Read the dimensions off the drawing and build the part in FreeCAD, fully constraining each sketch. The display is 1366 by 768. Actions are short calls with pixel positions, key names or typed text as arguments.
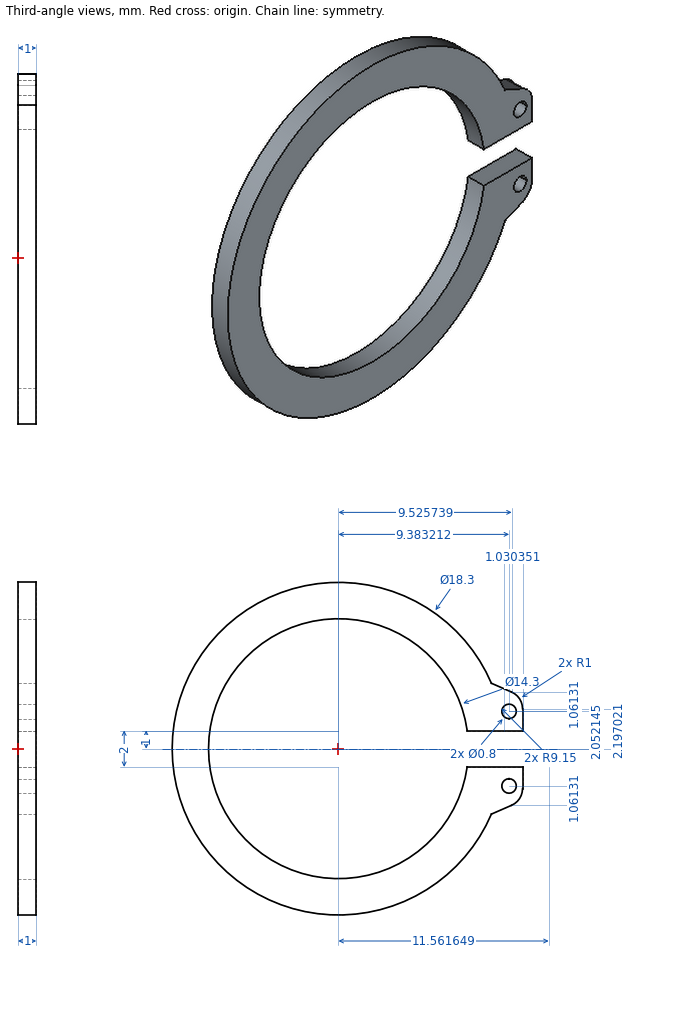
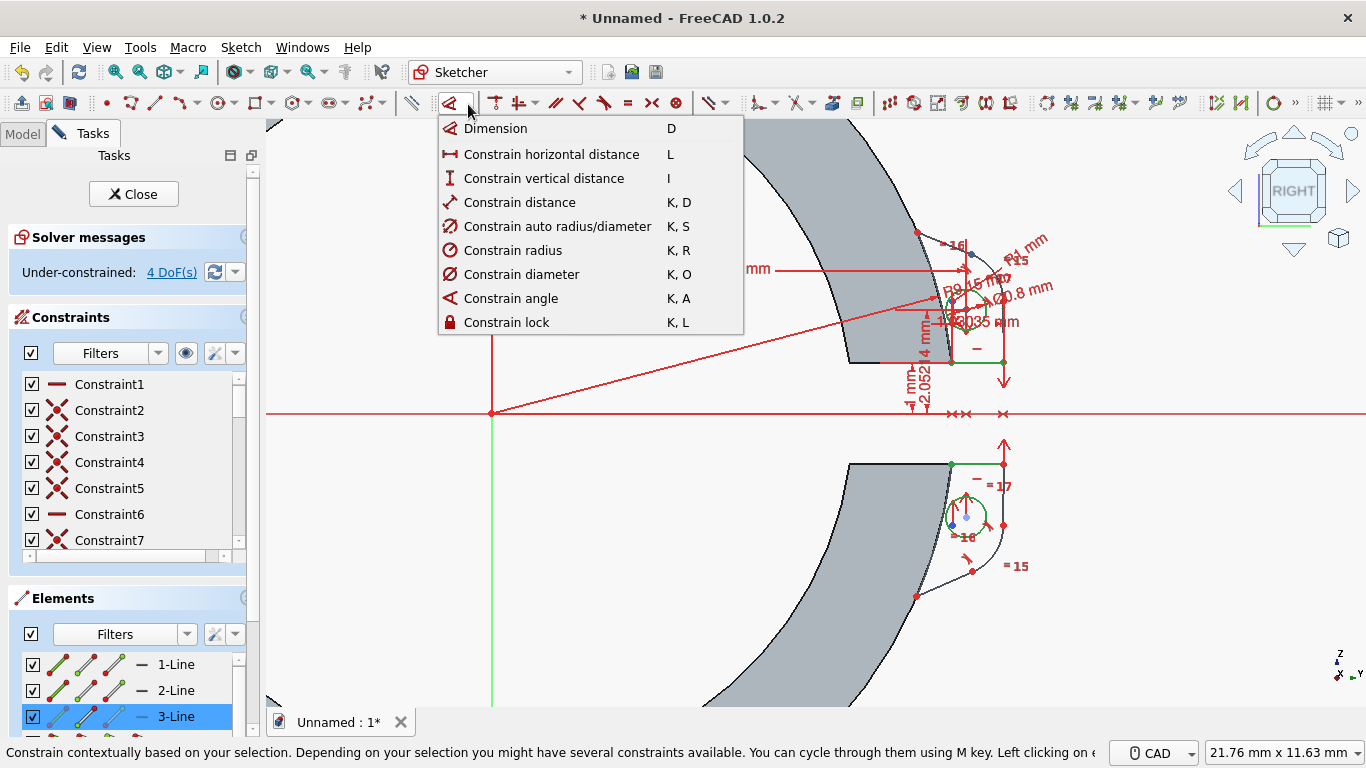
click(591, 178)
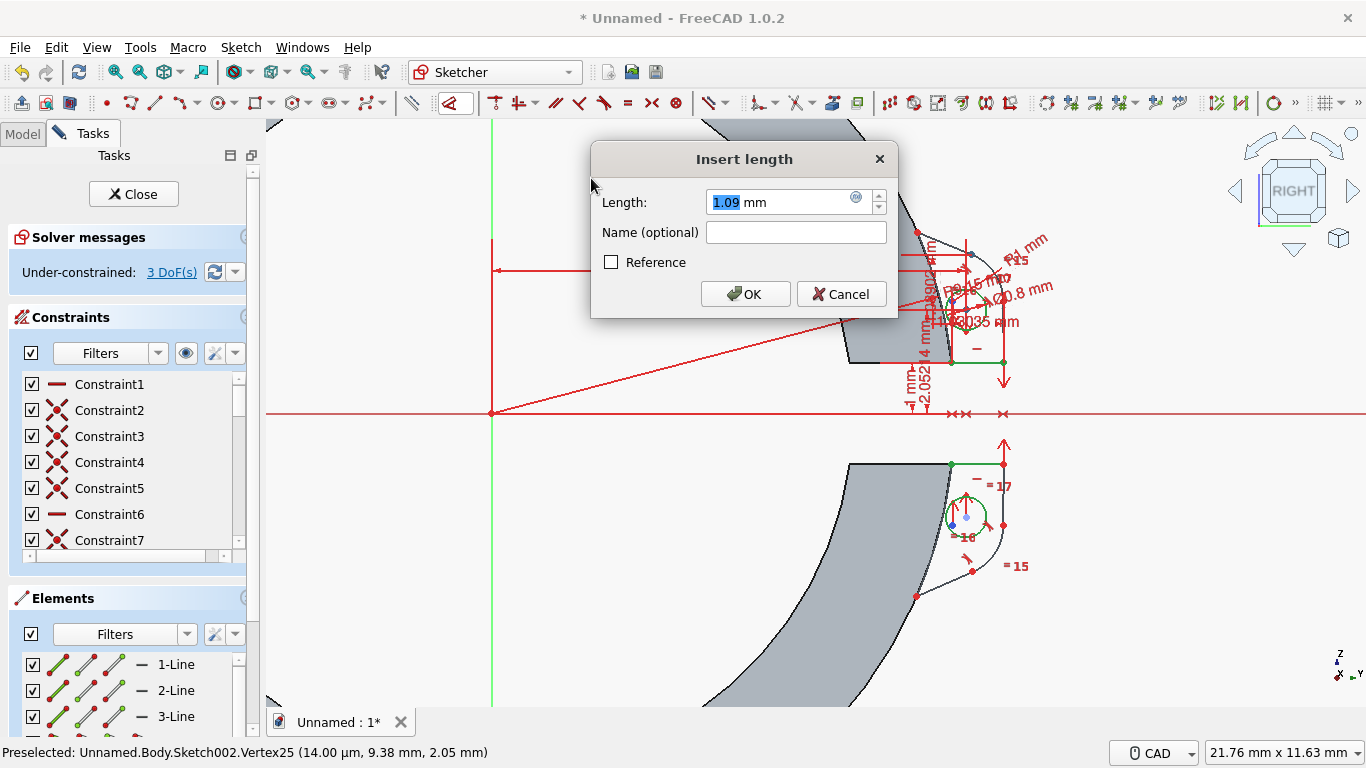
text(1.06131)
key(Return)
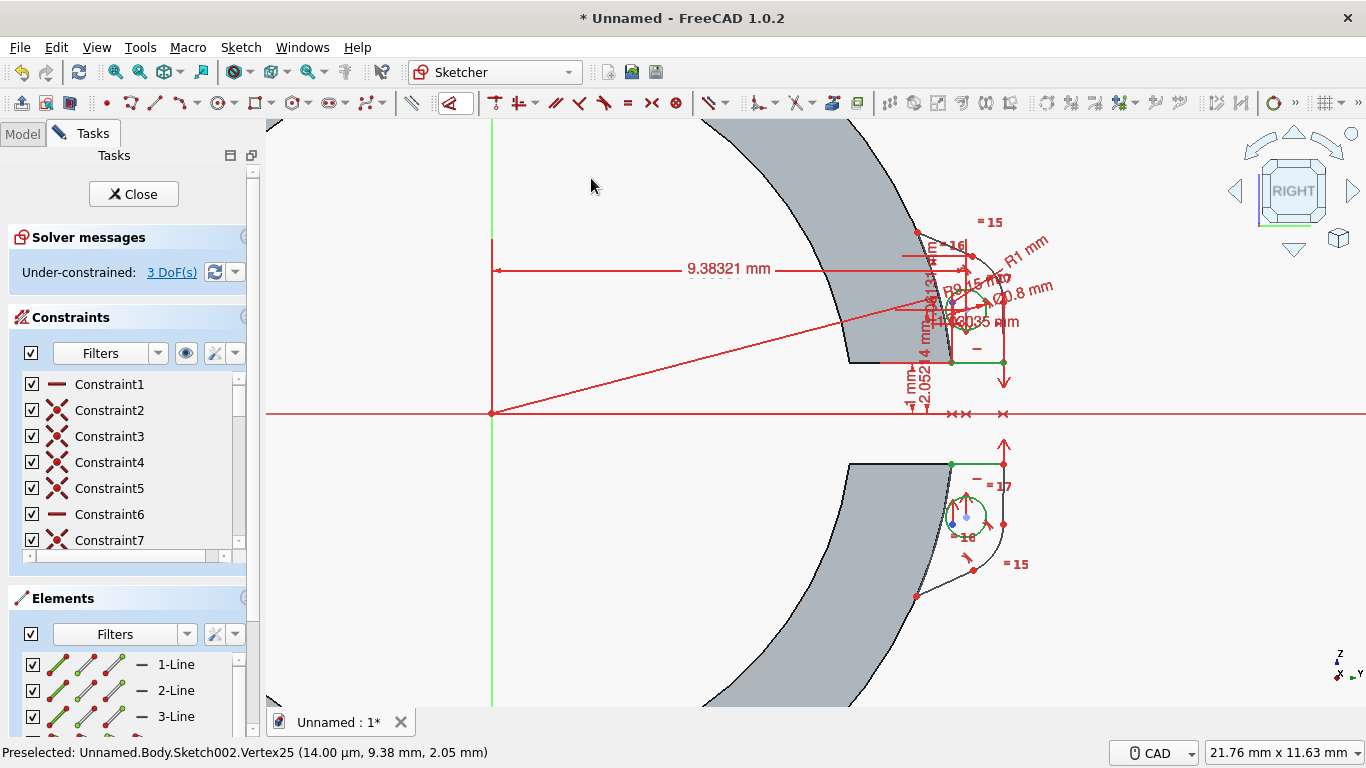
click(974, 570)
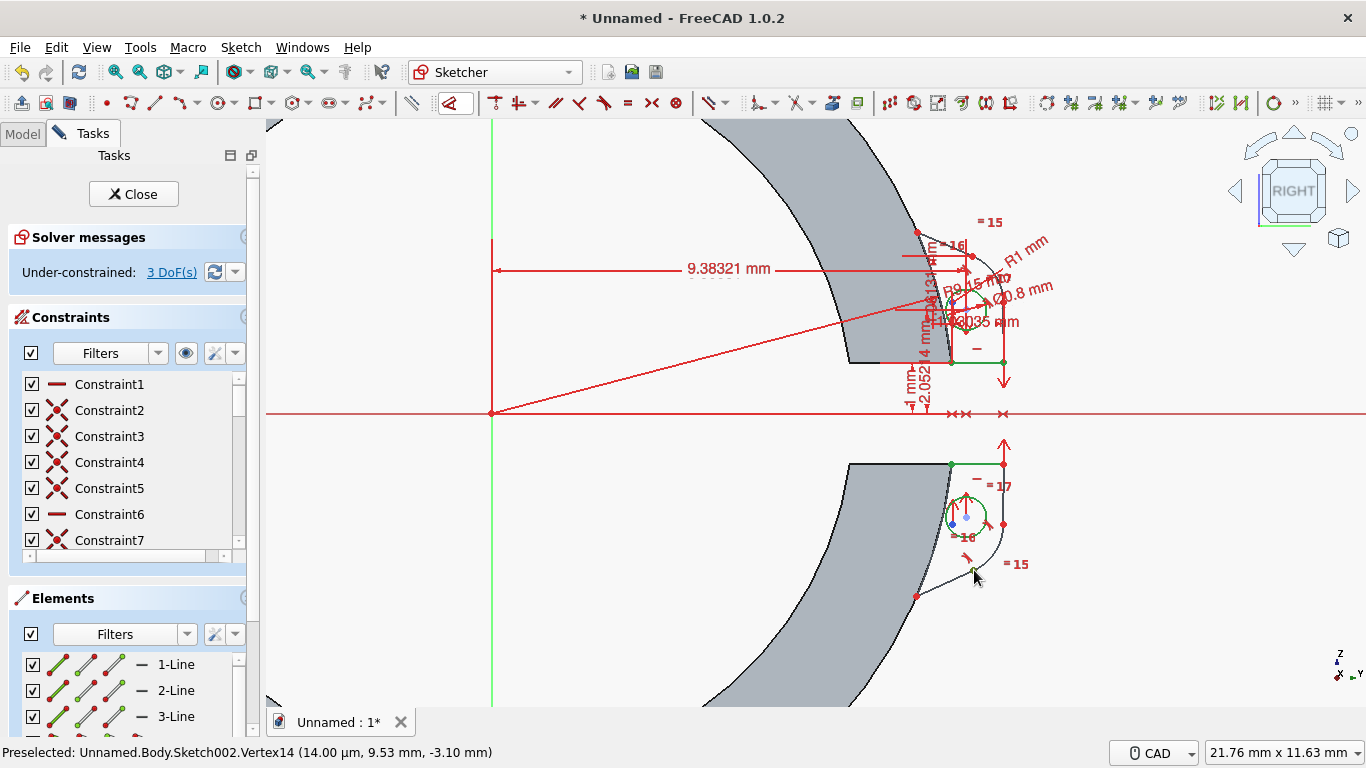
click(966, 517)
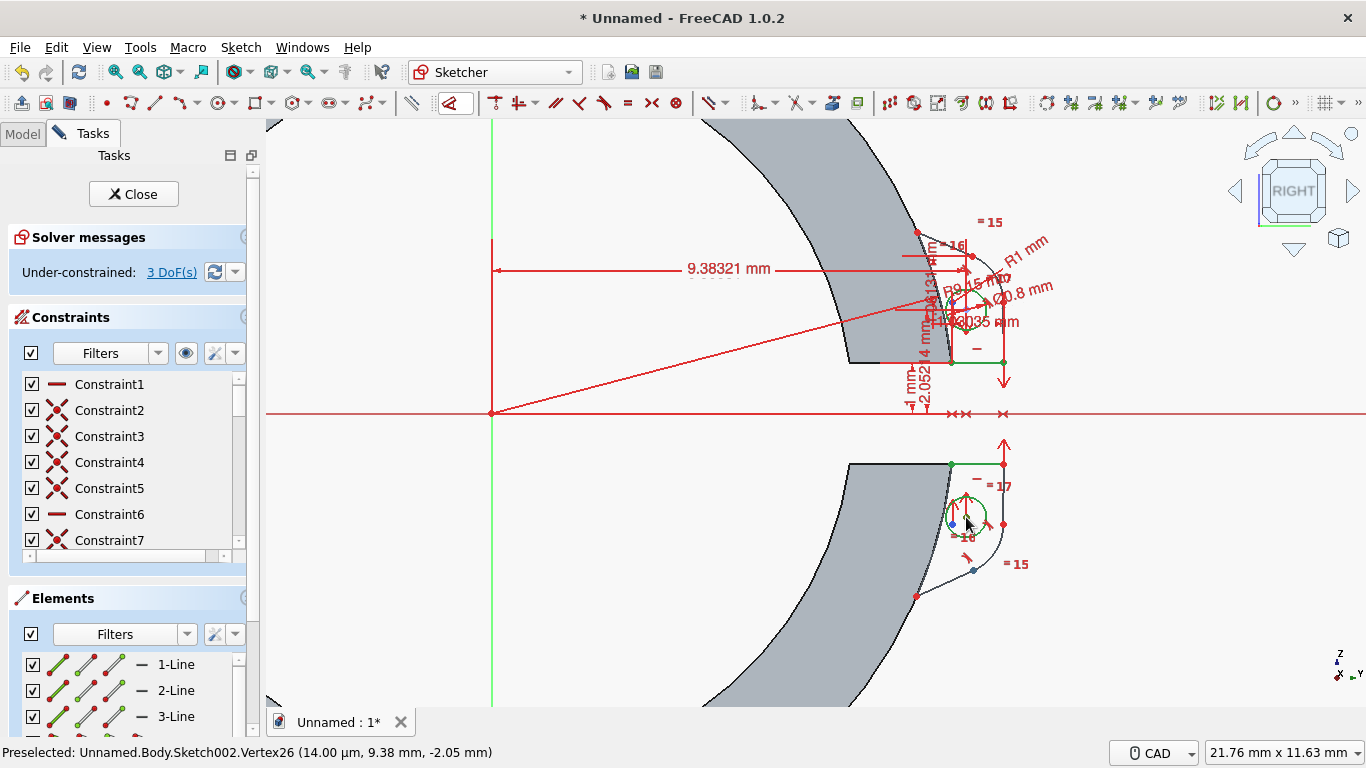
click(468, 104)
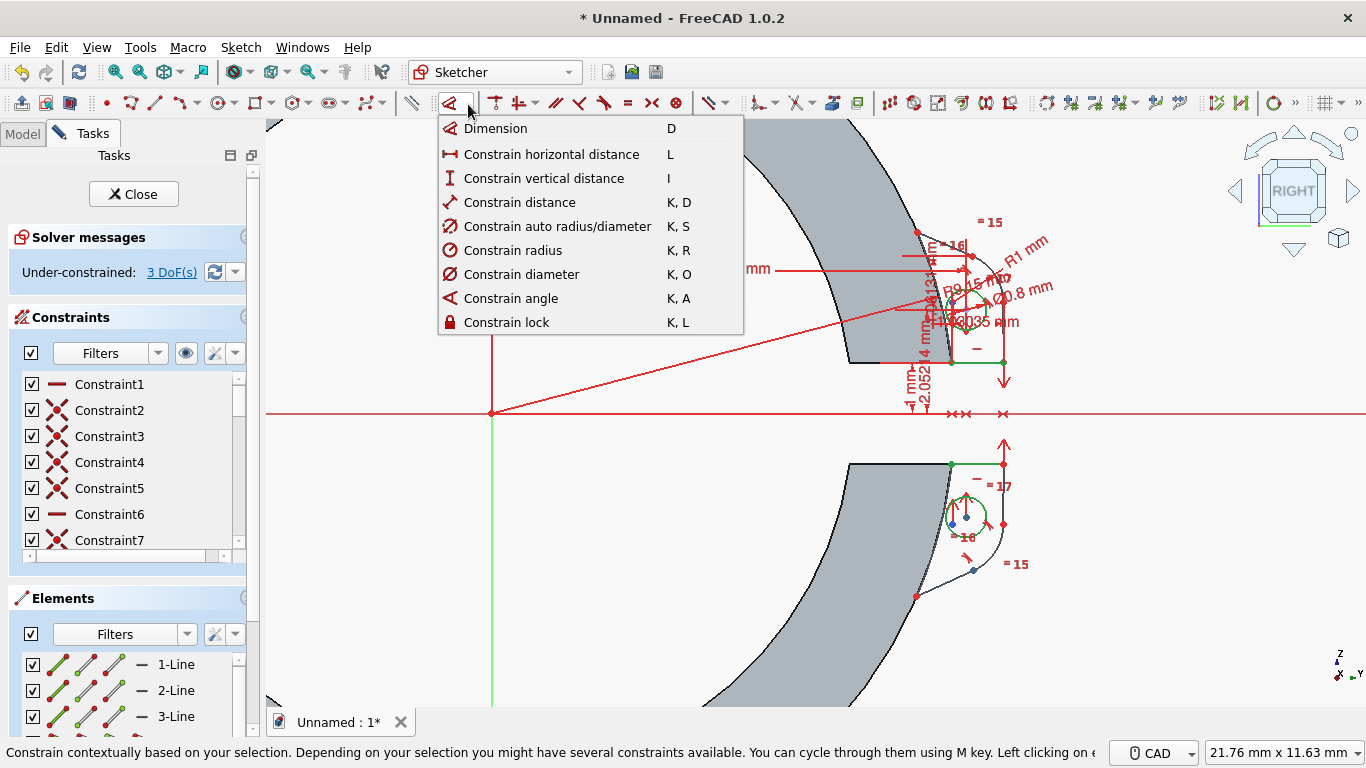
click(591, 178)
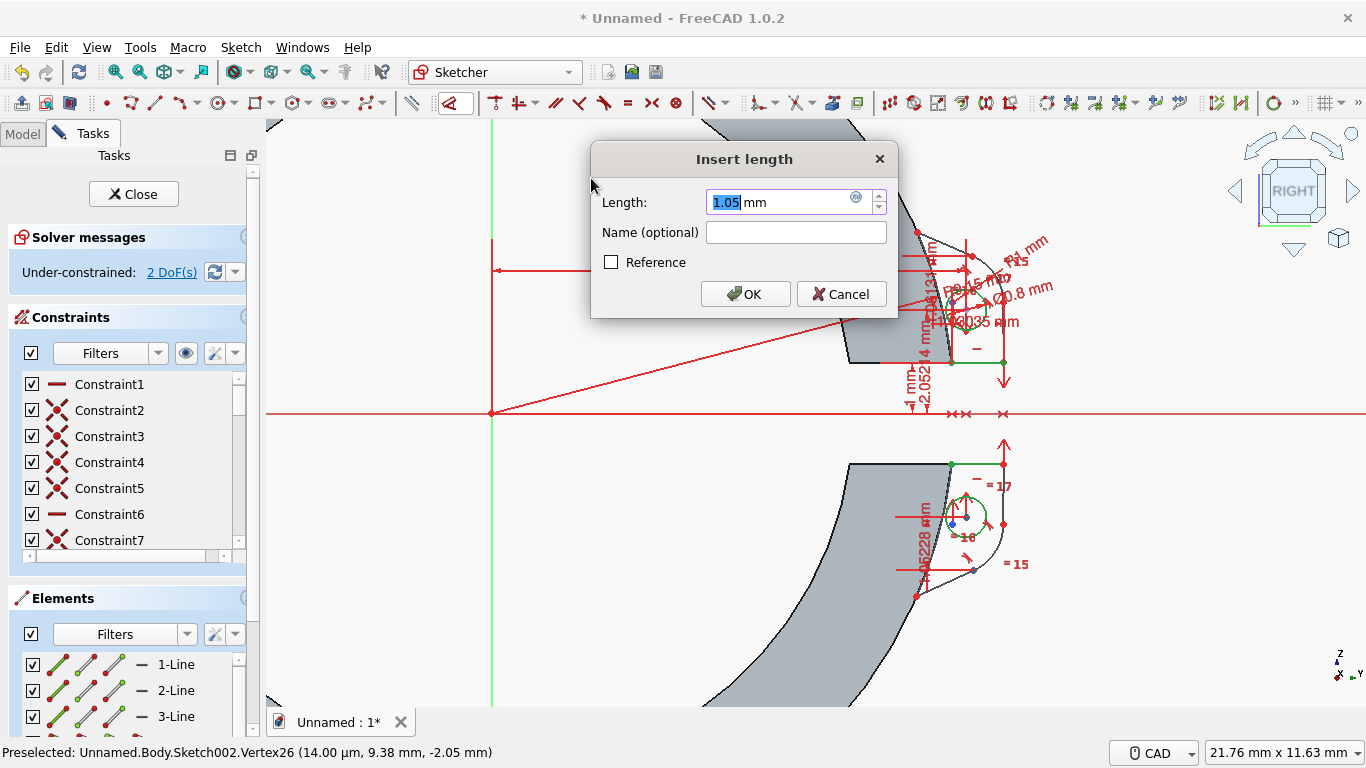
text(1.06131)
key(Return)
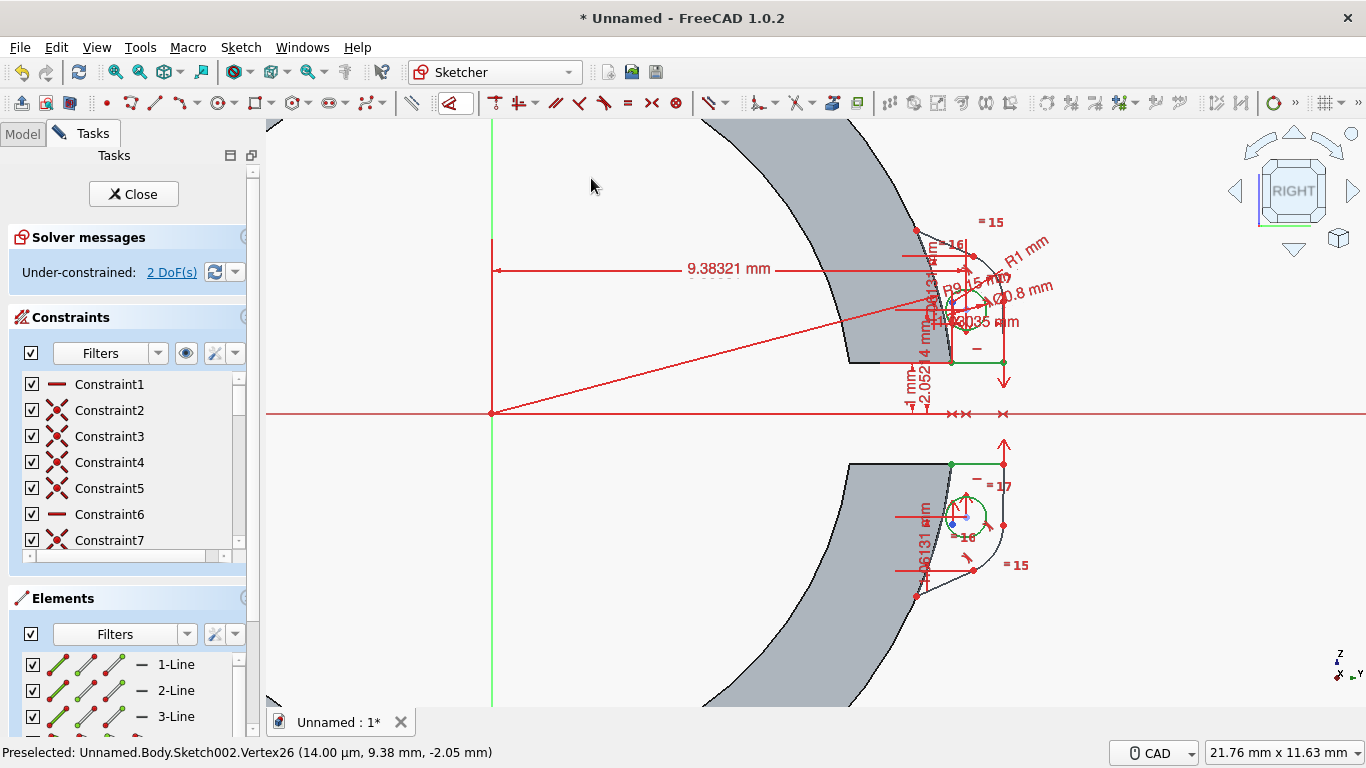
click(1003, 302)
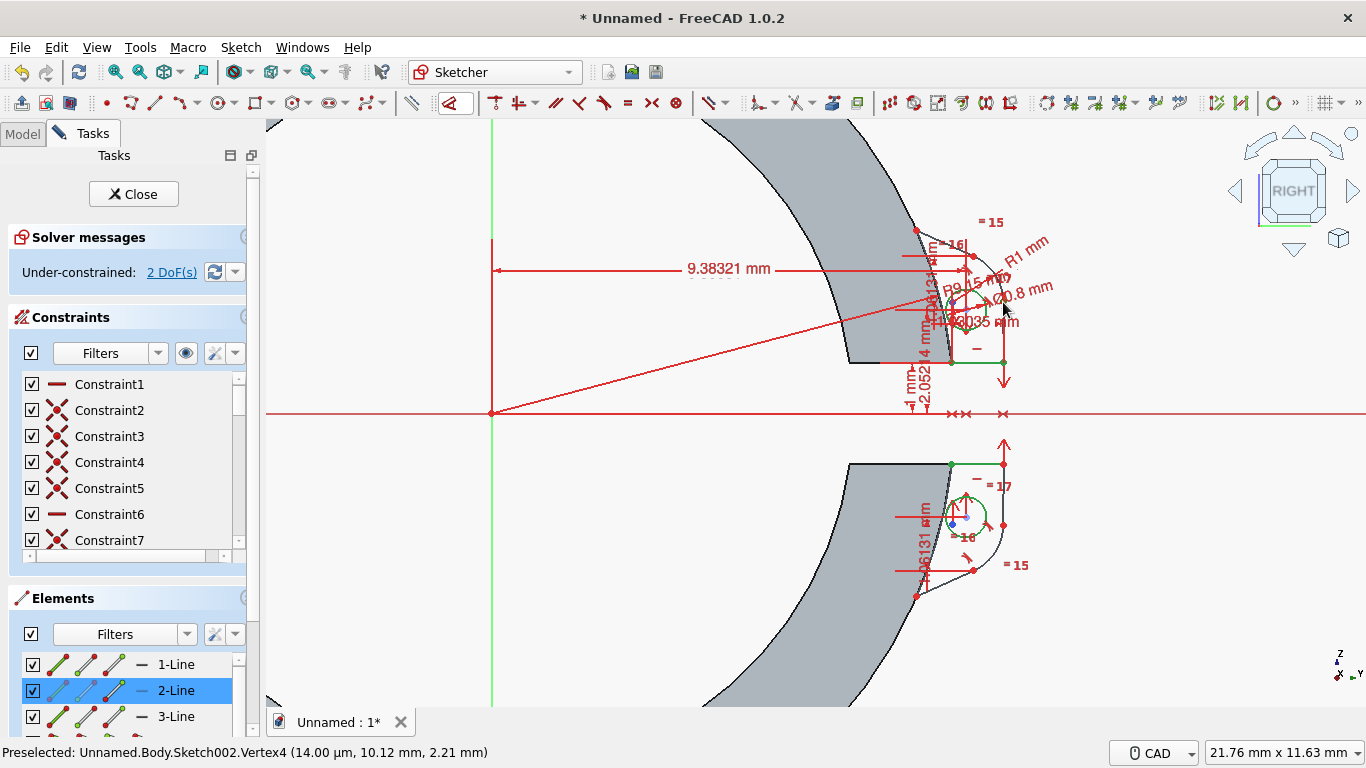
key(i)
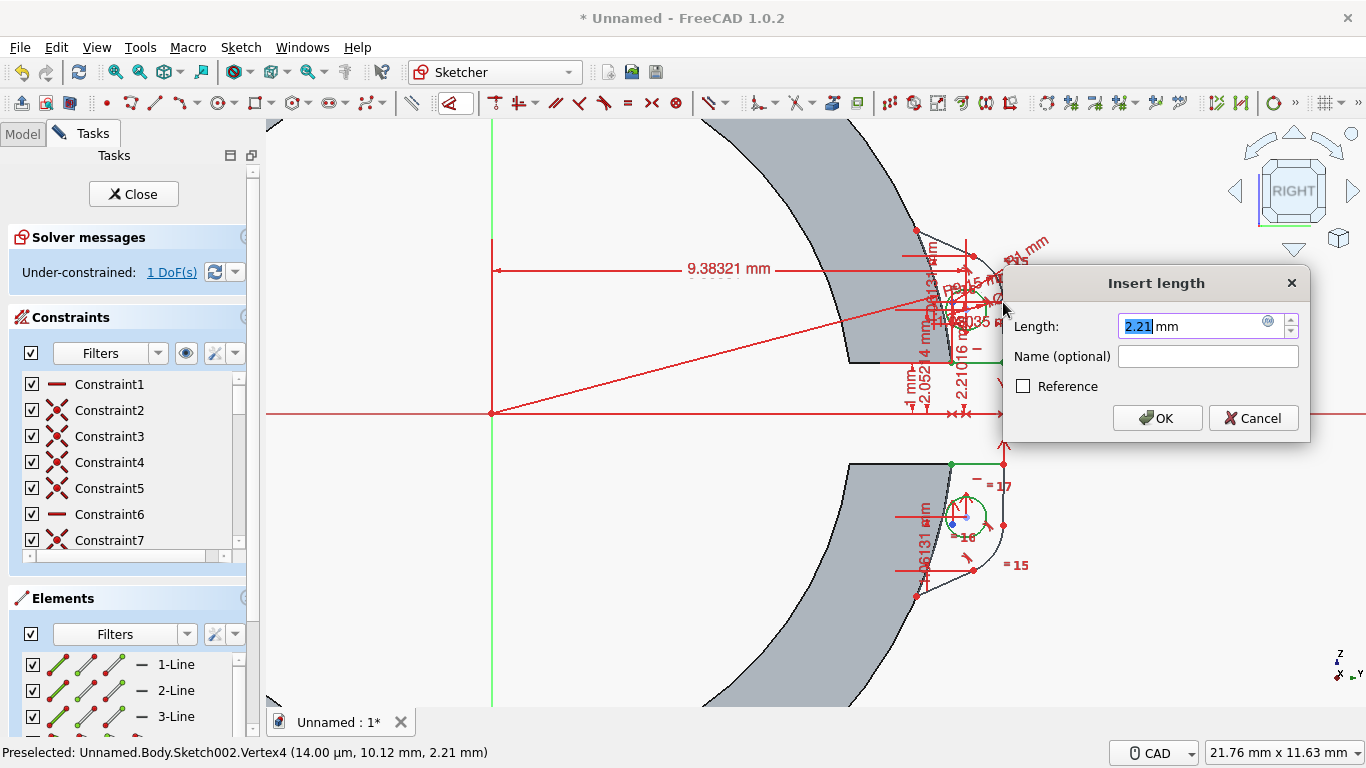
text(2.197021)
key(Return)